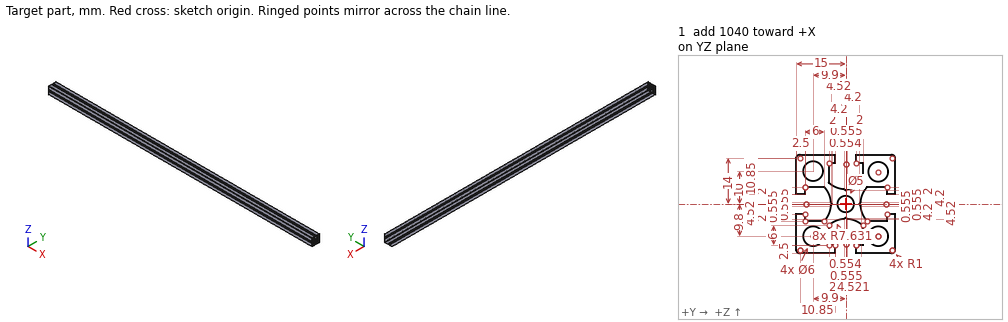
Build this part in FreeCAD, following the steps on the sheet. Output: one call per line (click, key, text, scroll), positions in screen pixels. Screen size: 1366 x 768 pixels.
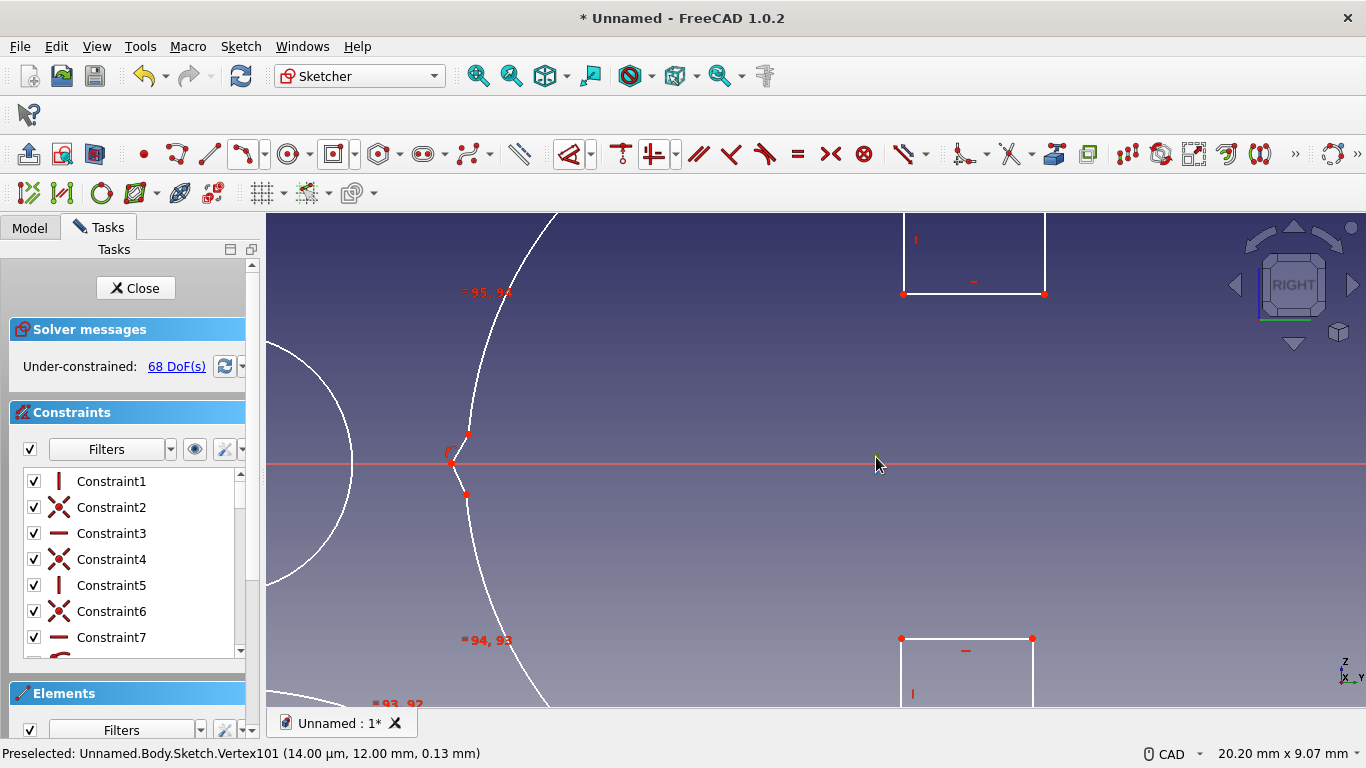
click(879, 470)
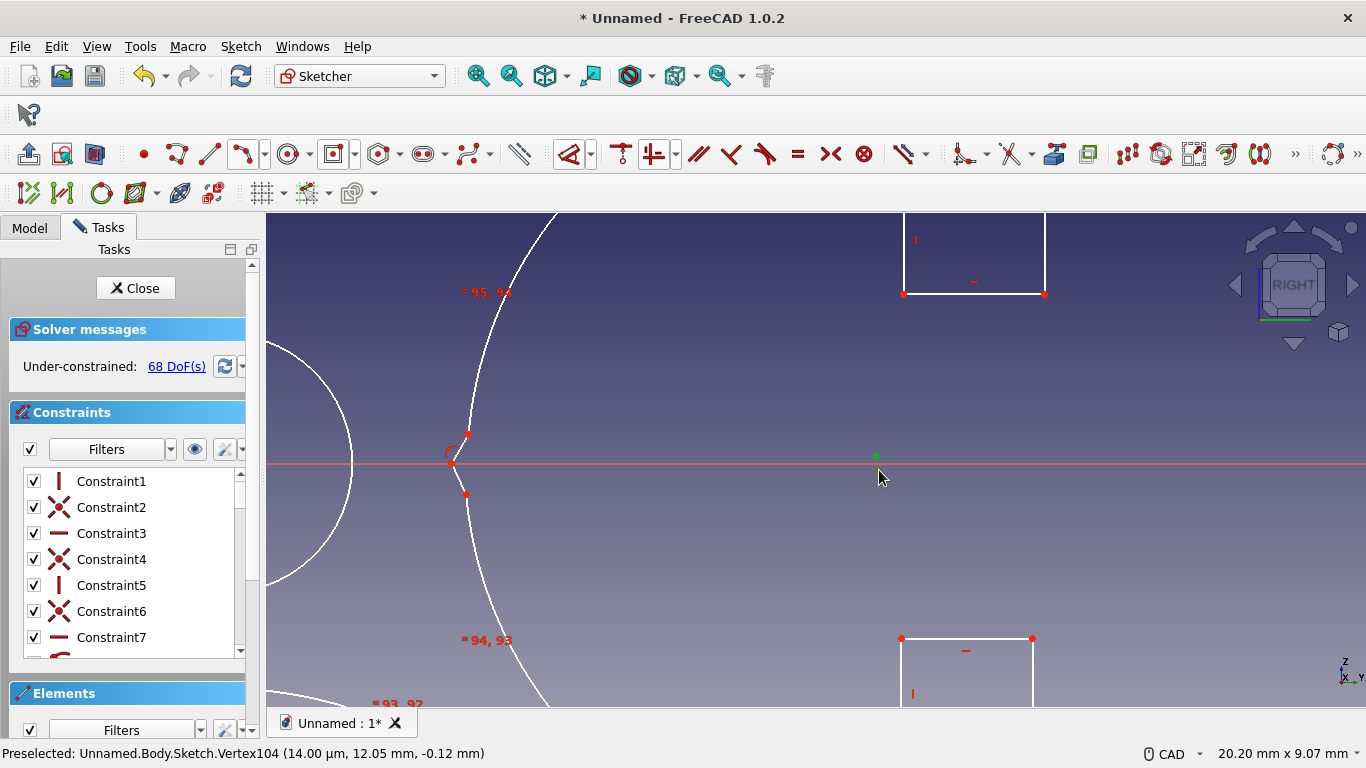
click(488, 464)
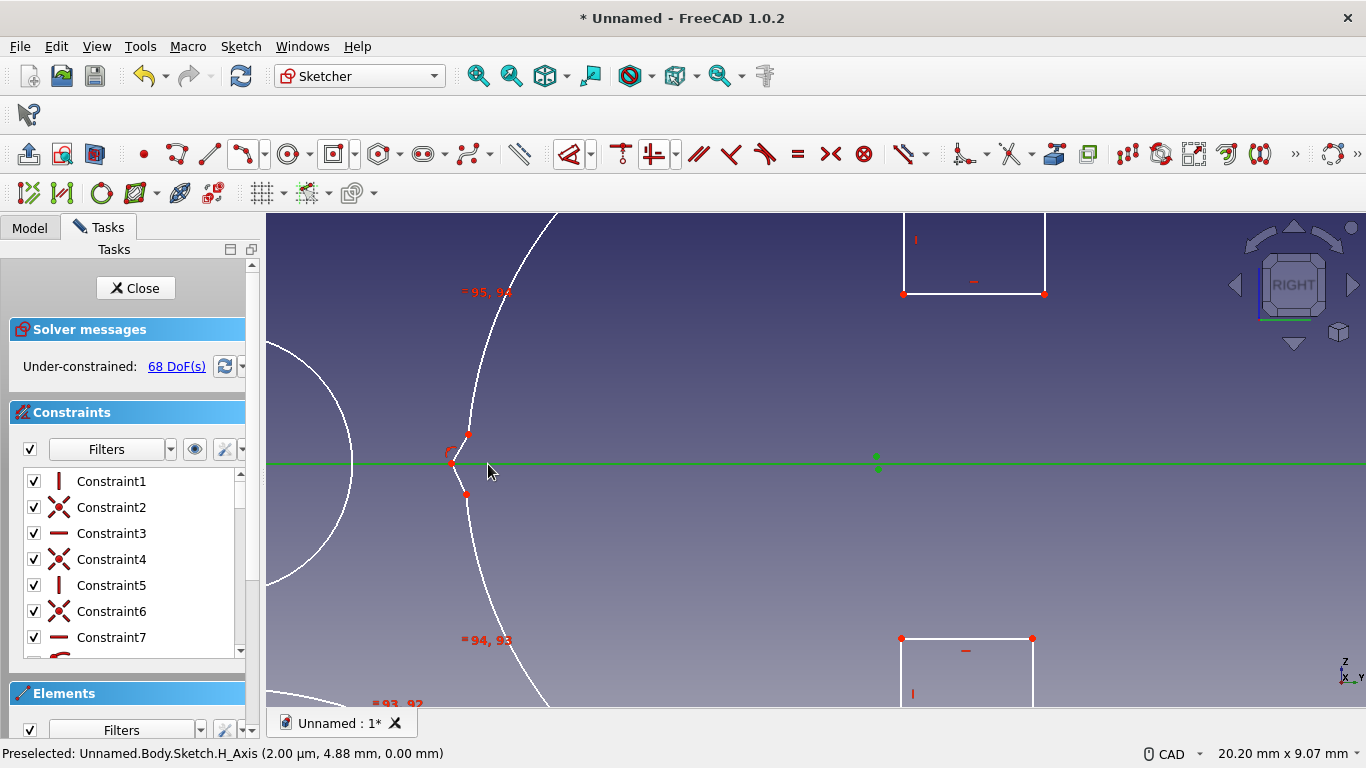
key(s)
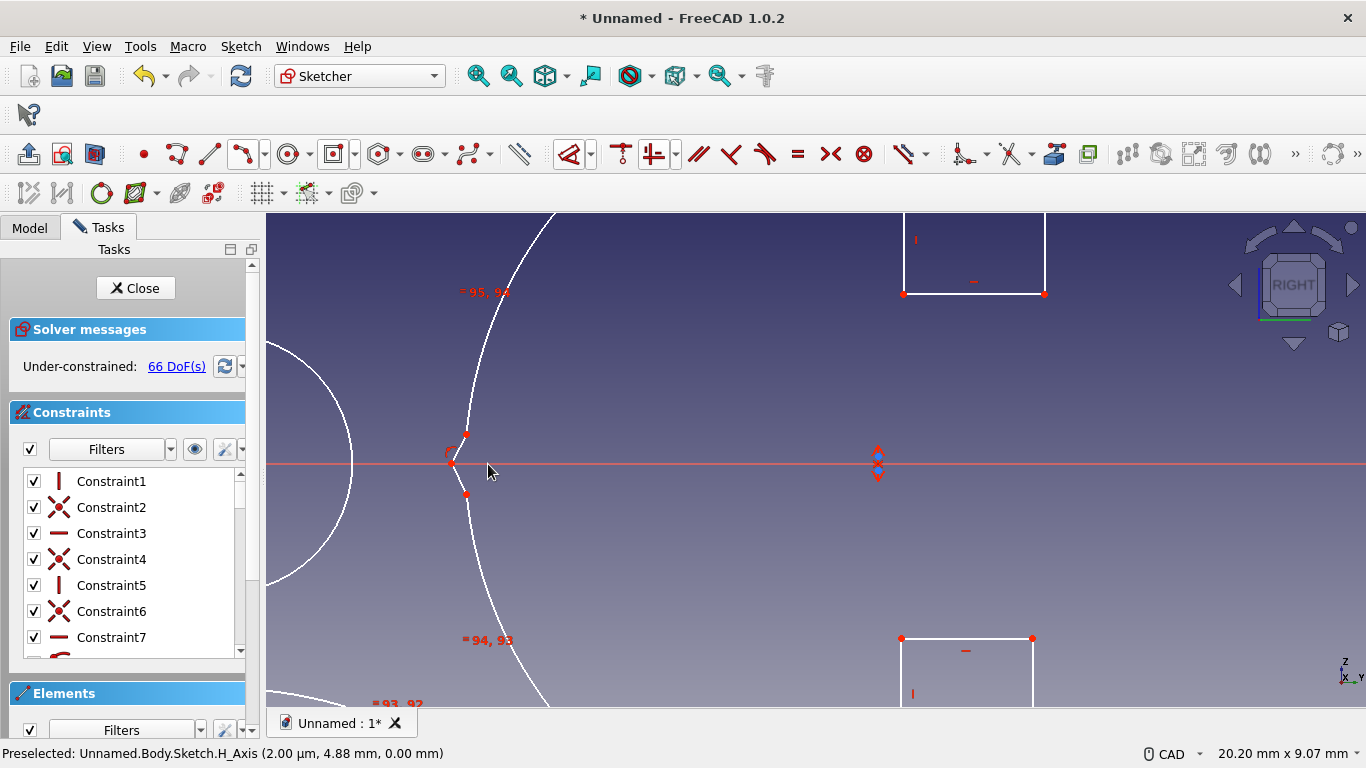
scroll(880, 459, down, 8)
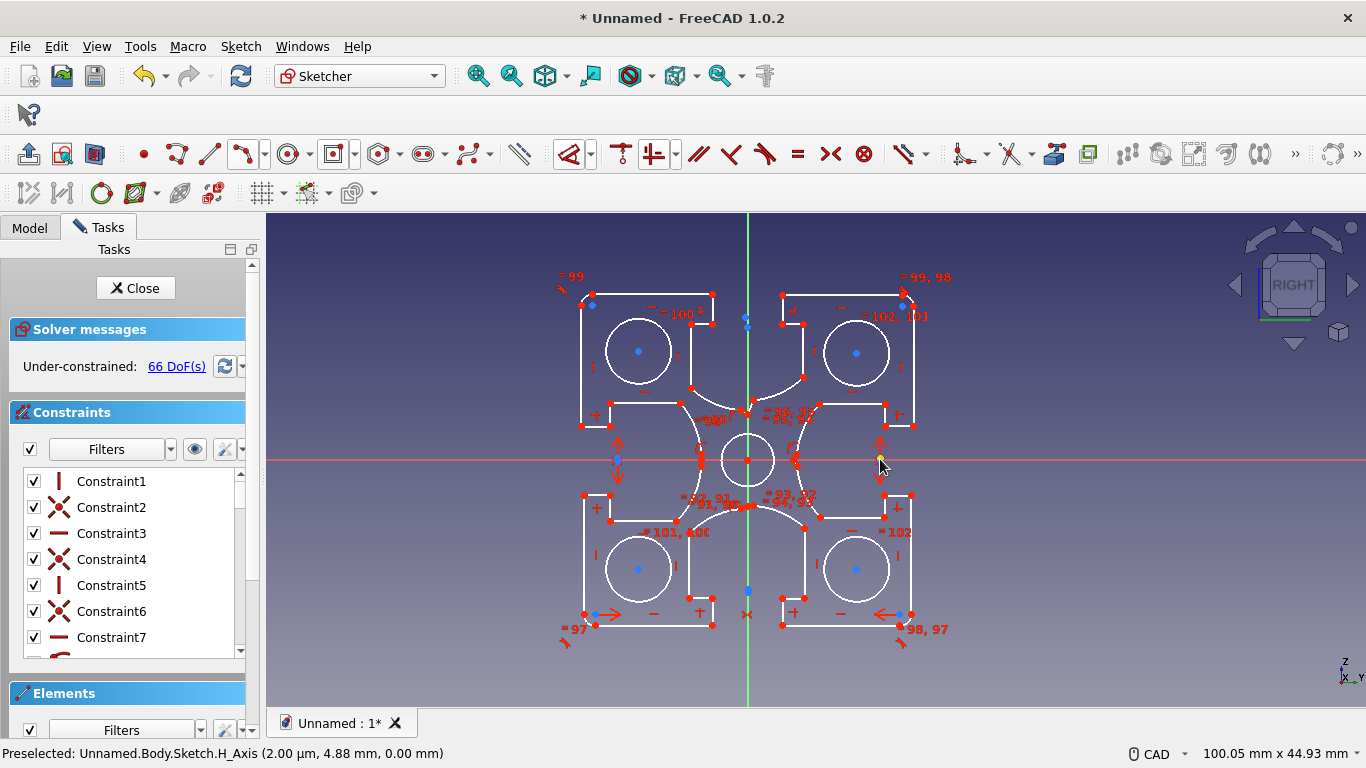
click(900, 615)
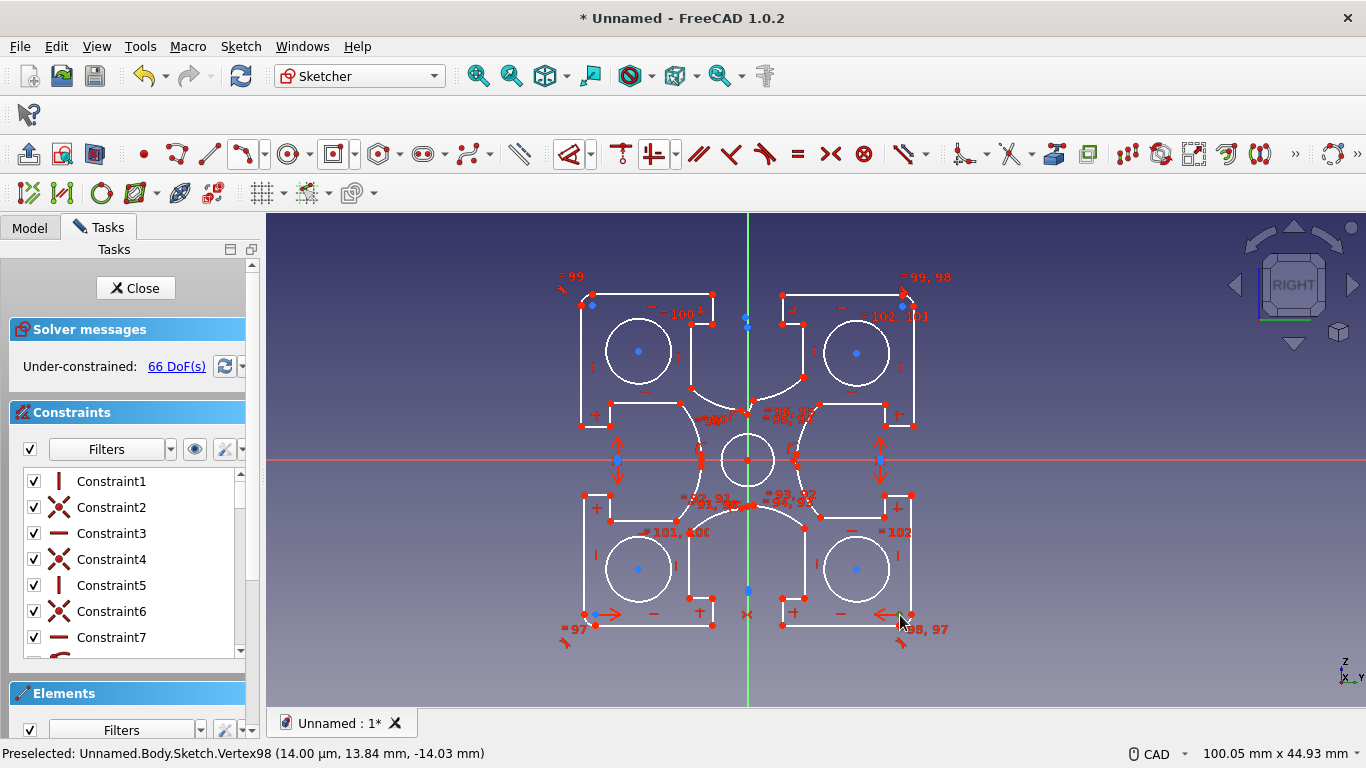
click(902, 306)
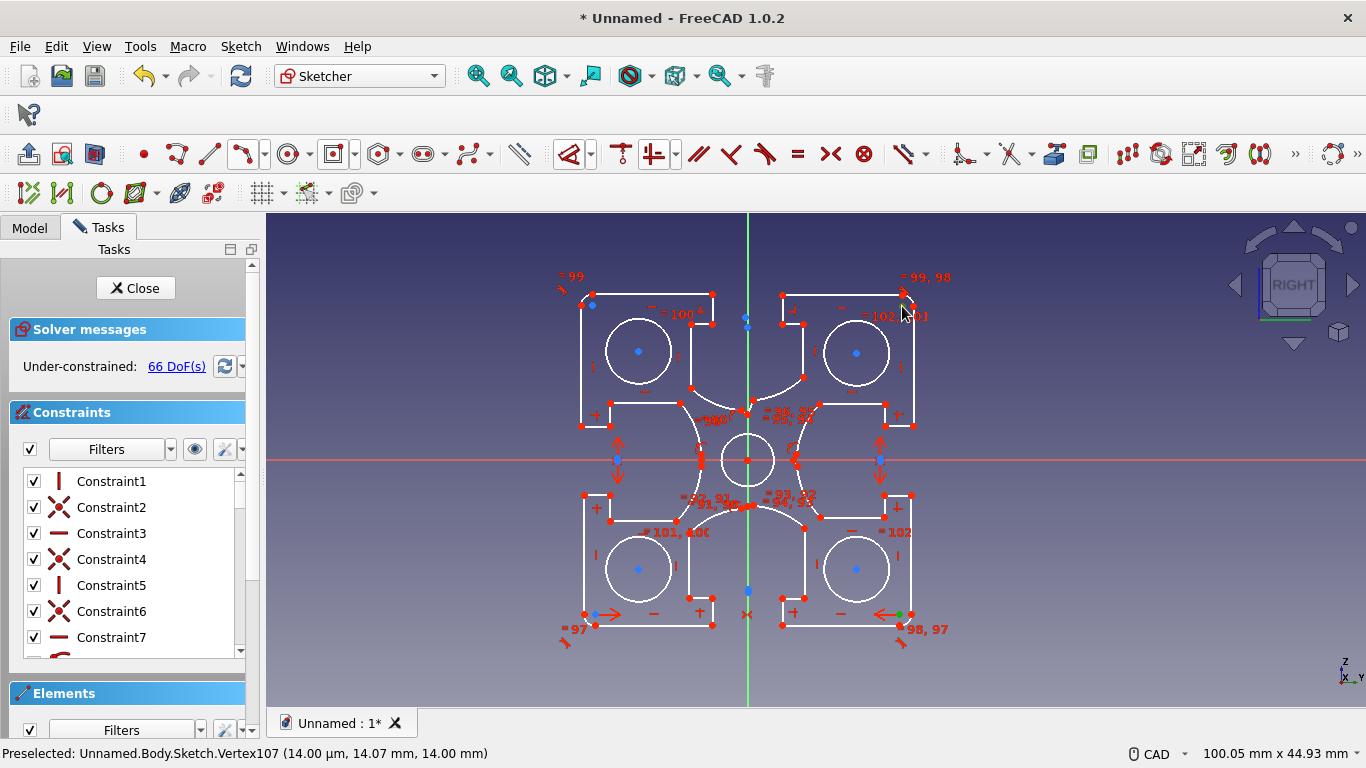
click(359, 460)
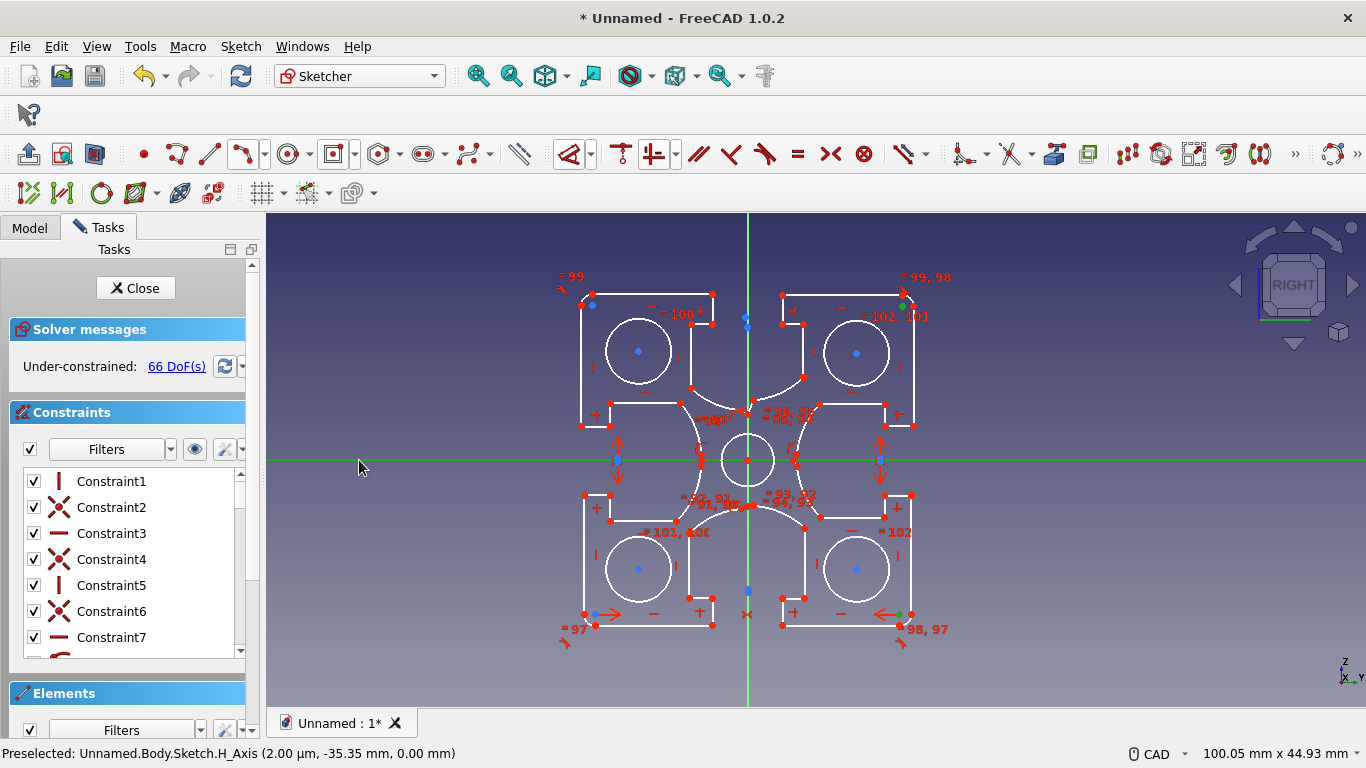
key(s)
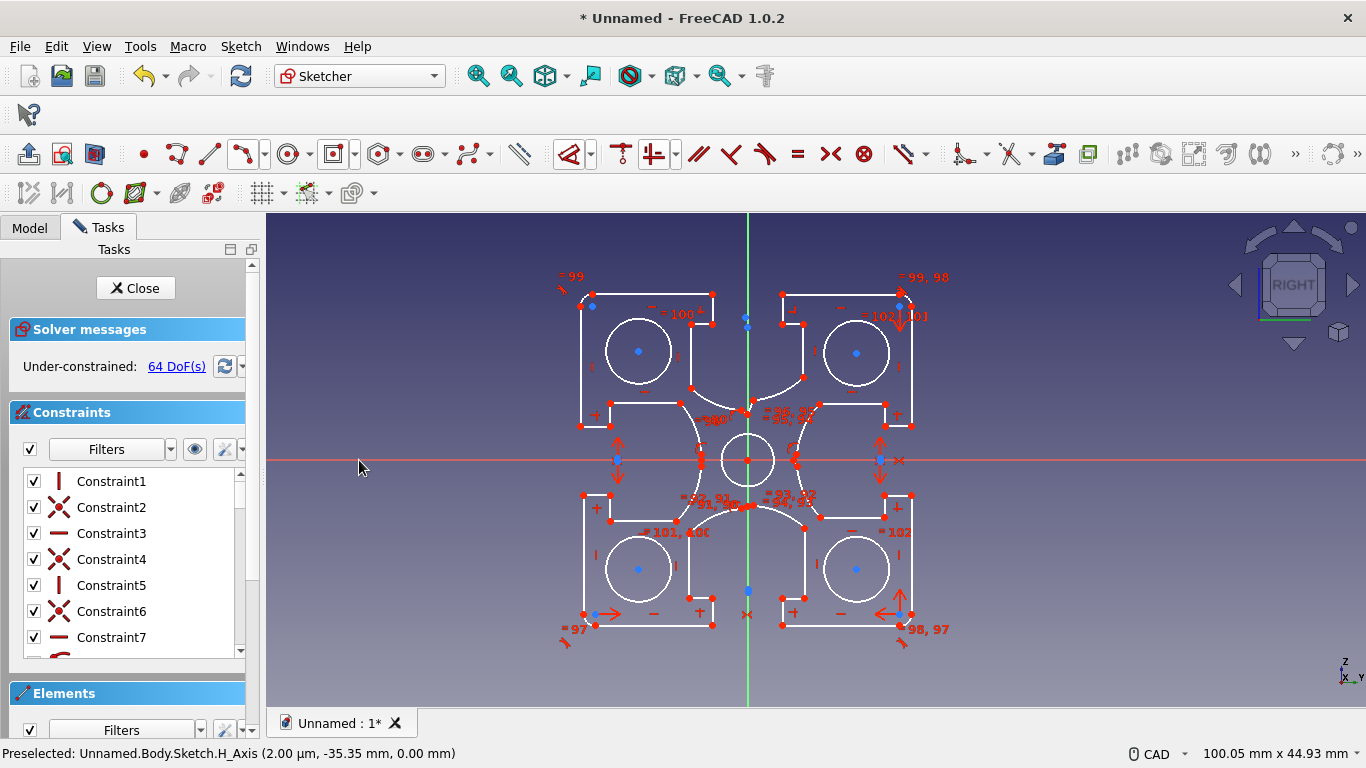
scroll(748, 589, up, 8)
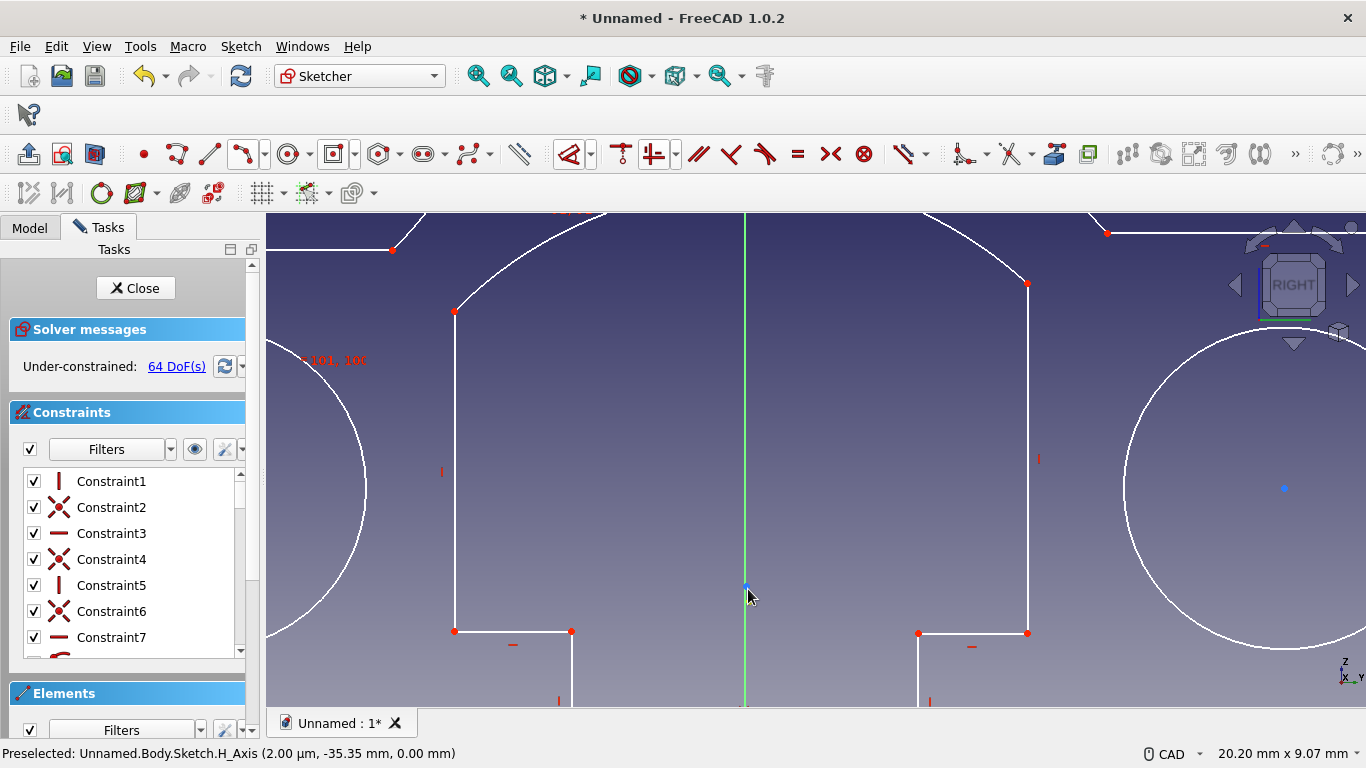
click(747, 587)